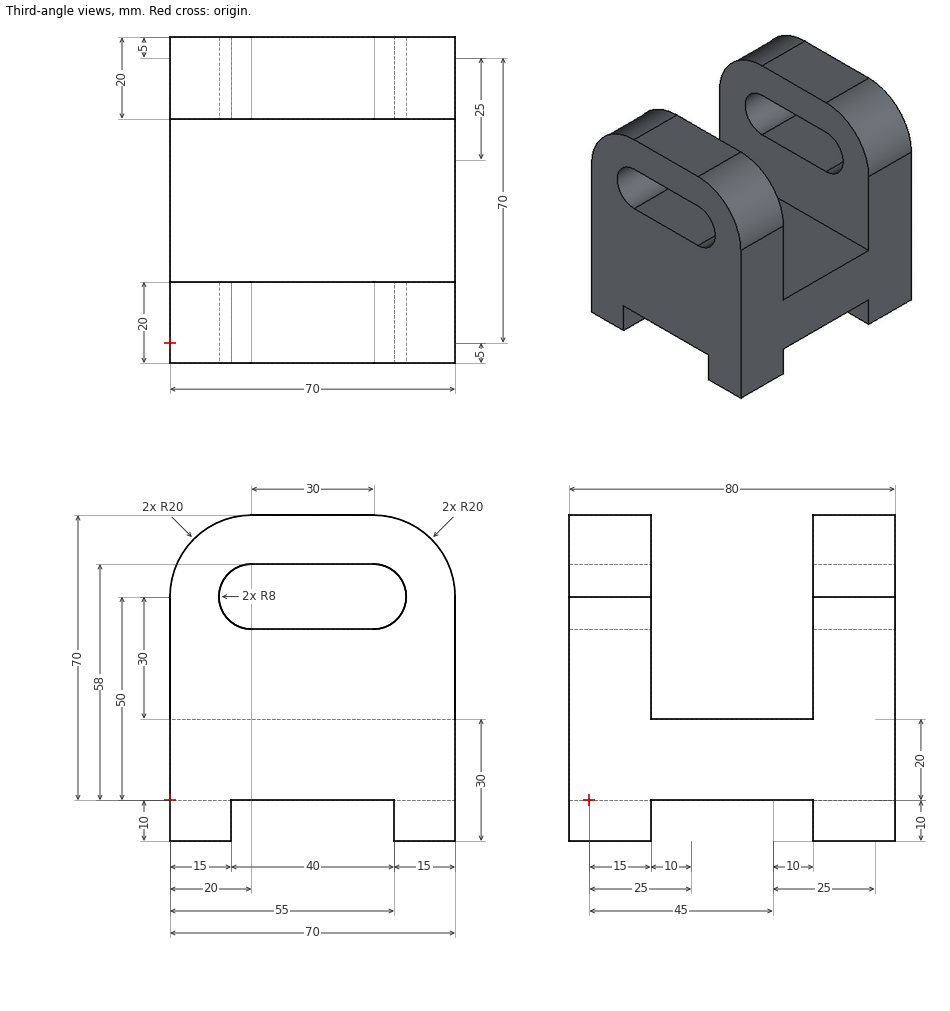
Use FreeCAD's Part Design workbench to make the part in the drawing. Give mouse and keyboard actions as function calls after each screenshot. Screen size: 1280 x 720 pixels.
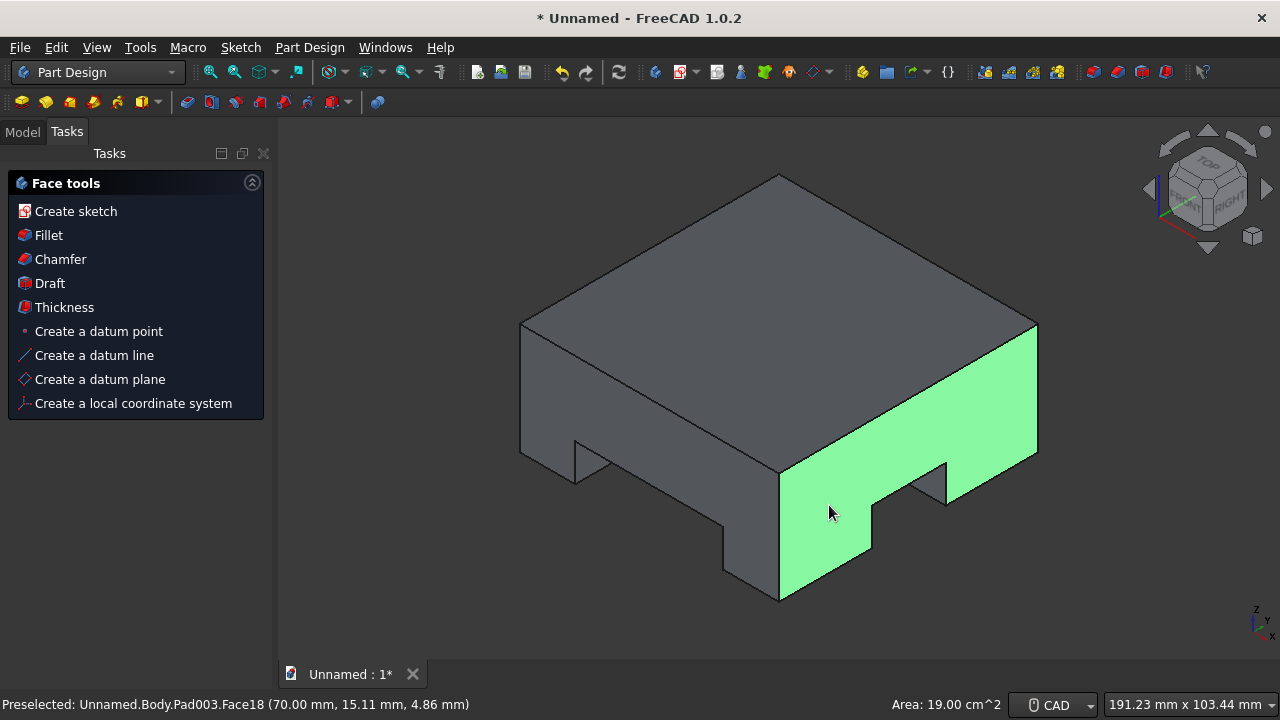
click(680, 72)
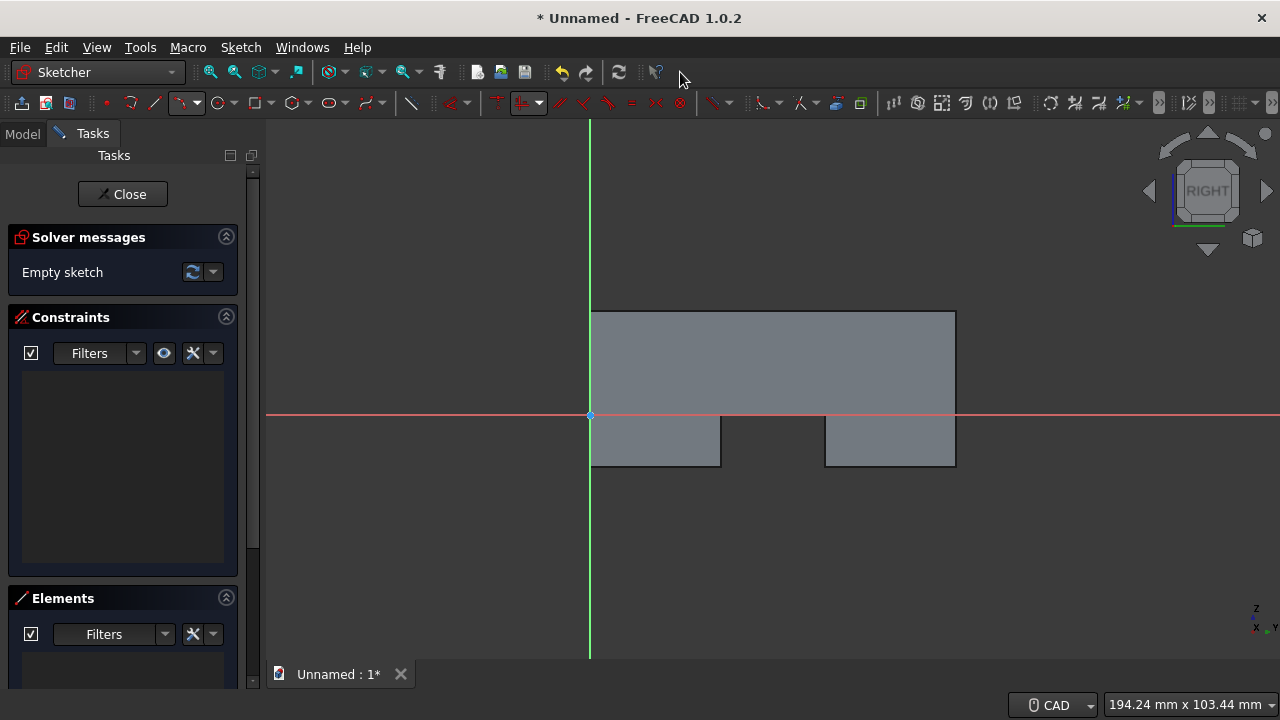
scroll(880, 452, up, 9)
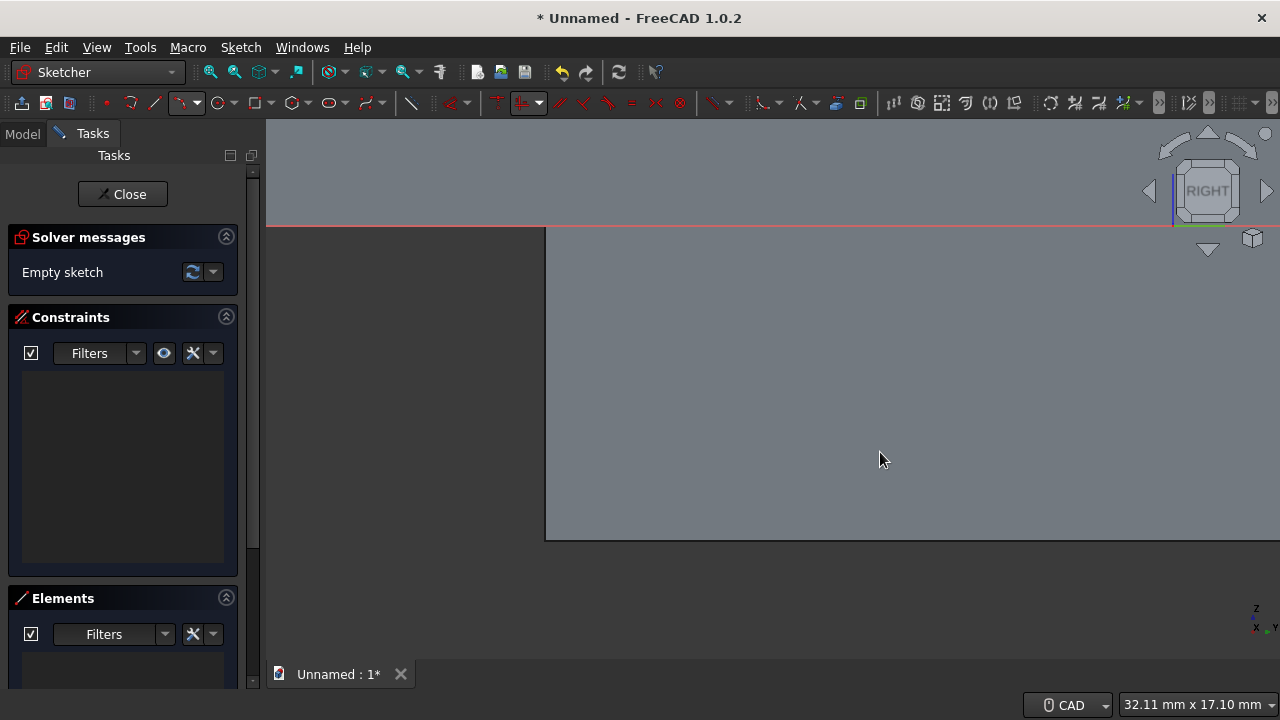
key(g)
key(r)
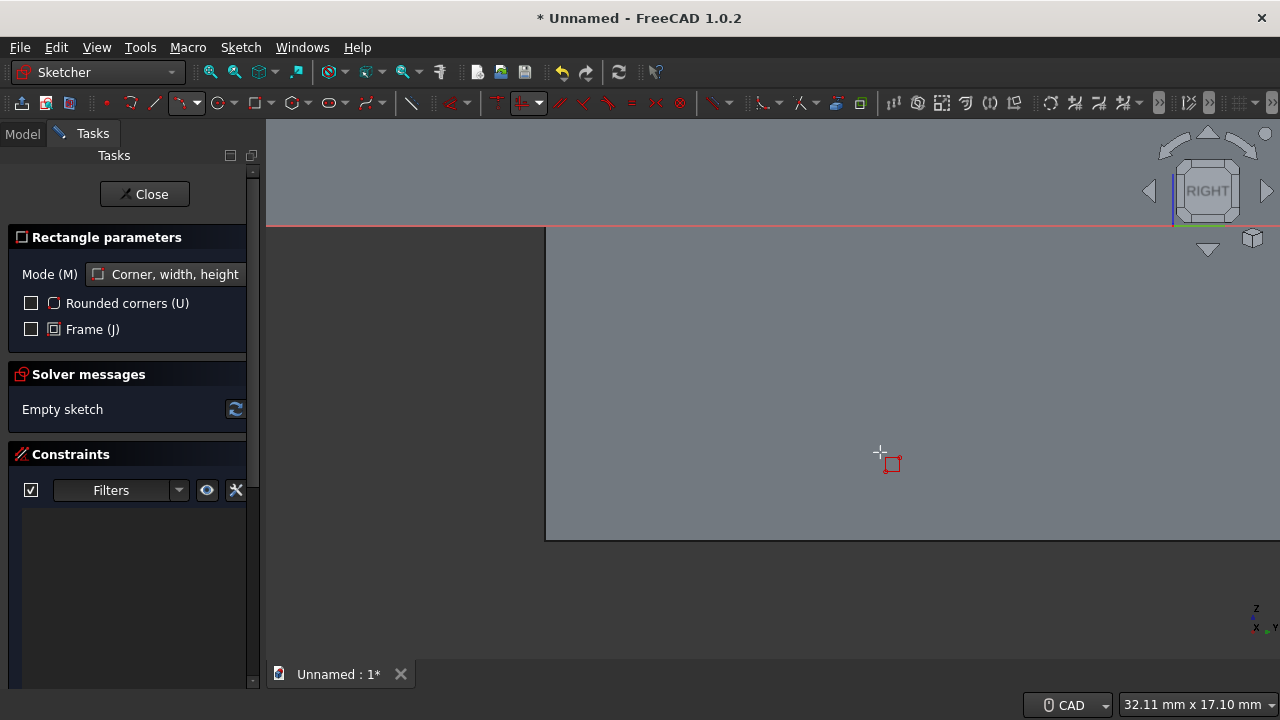
click(545, 226)
click(861, 541)
key(Escape)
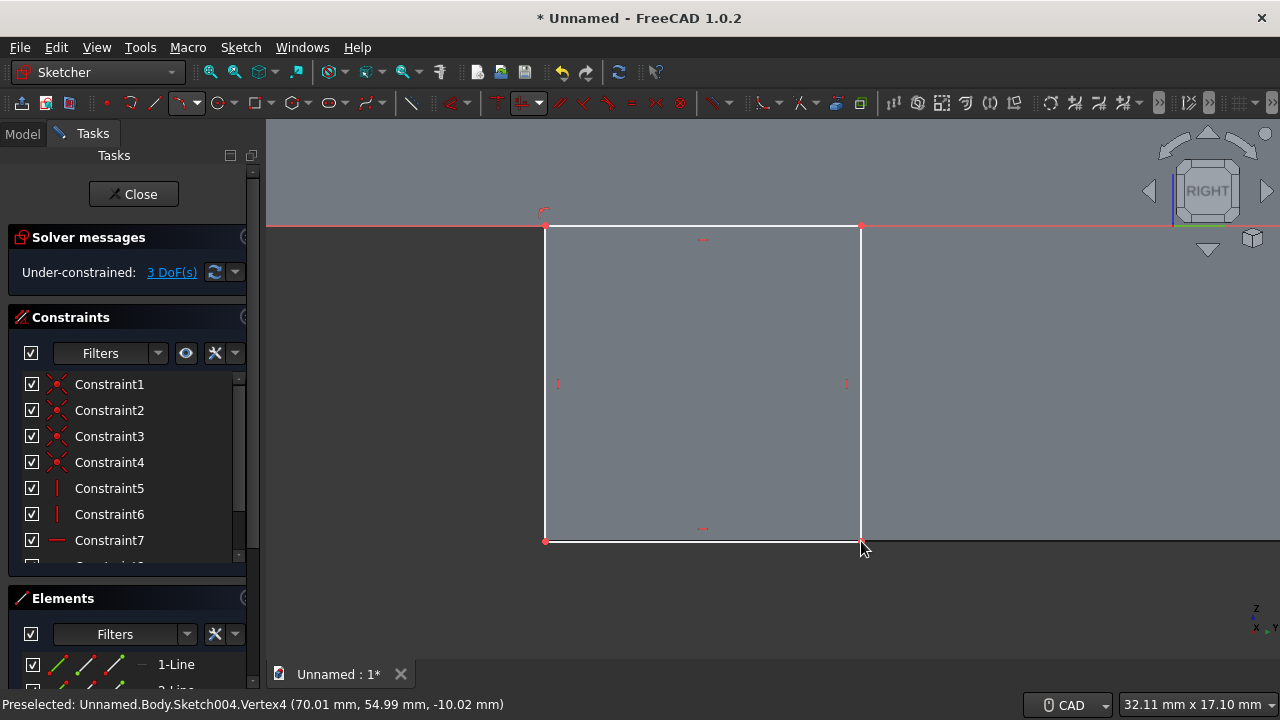
key(d)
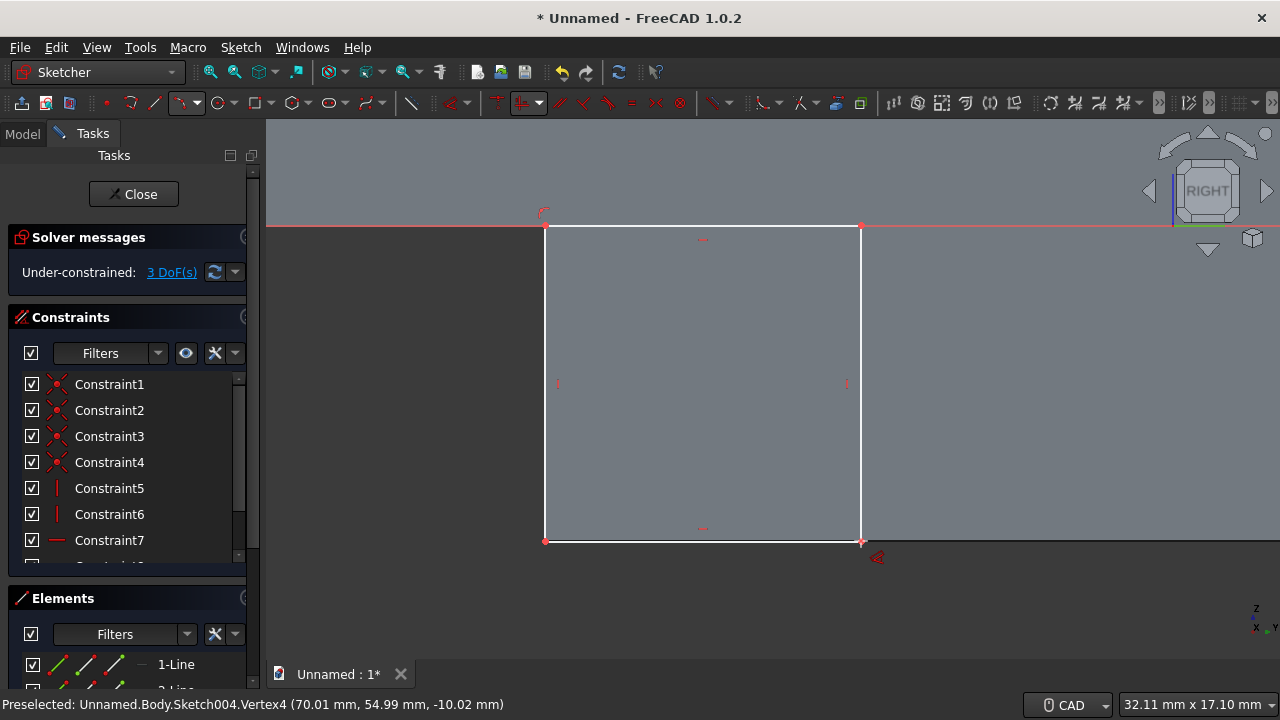
click(545, 321)
click(511, 384)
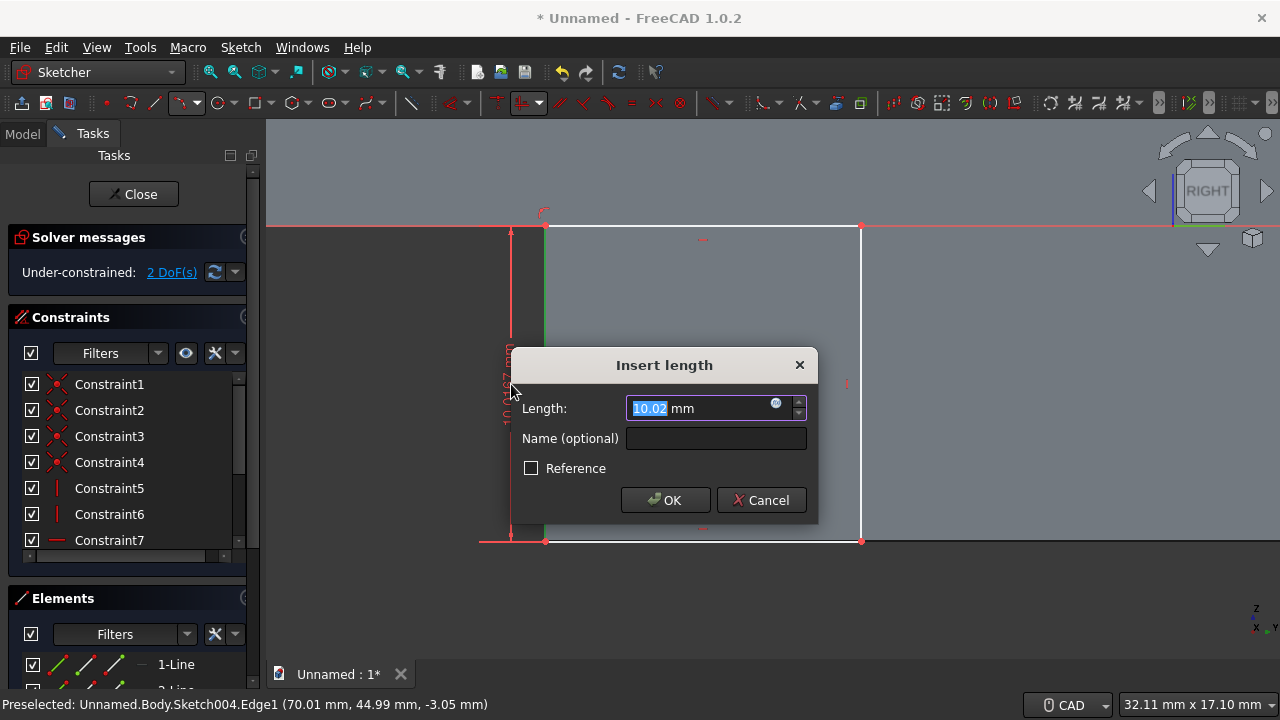
text(10)
key(Return)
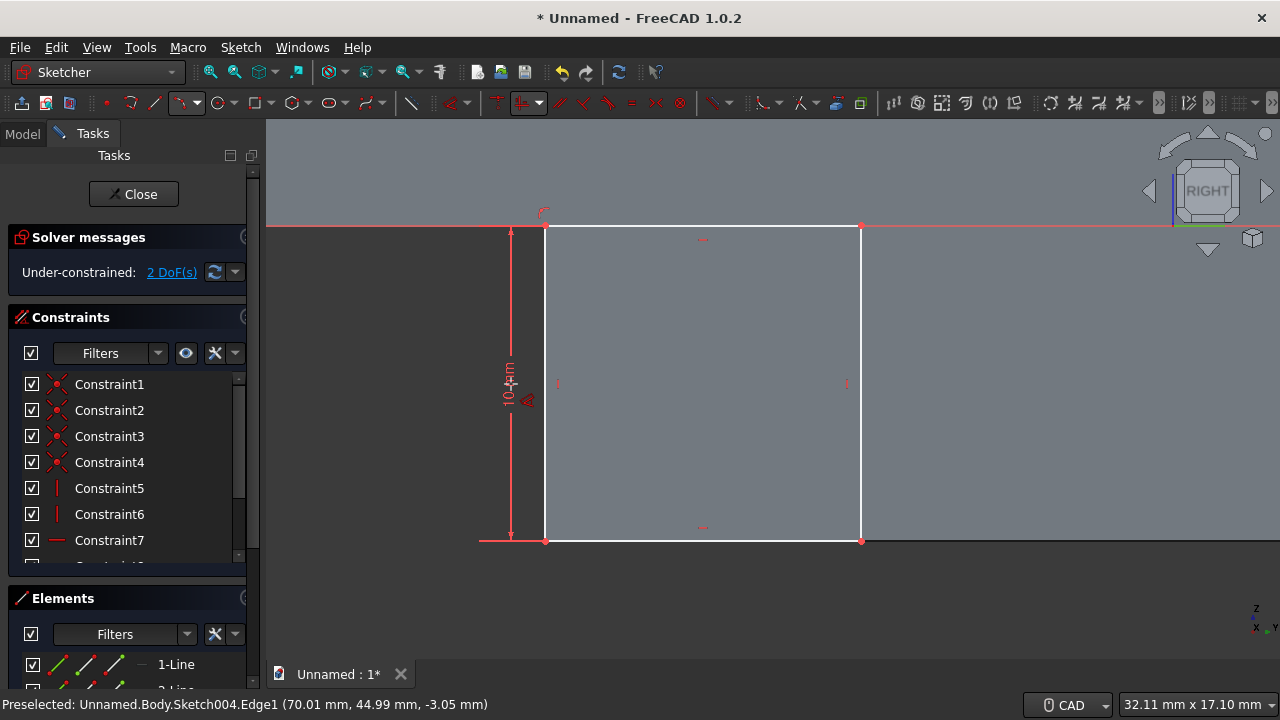
click(640, 541)
click(703, 575)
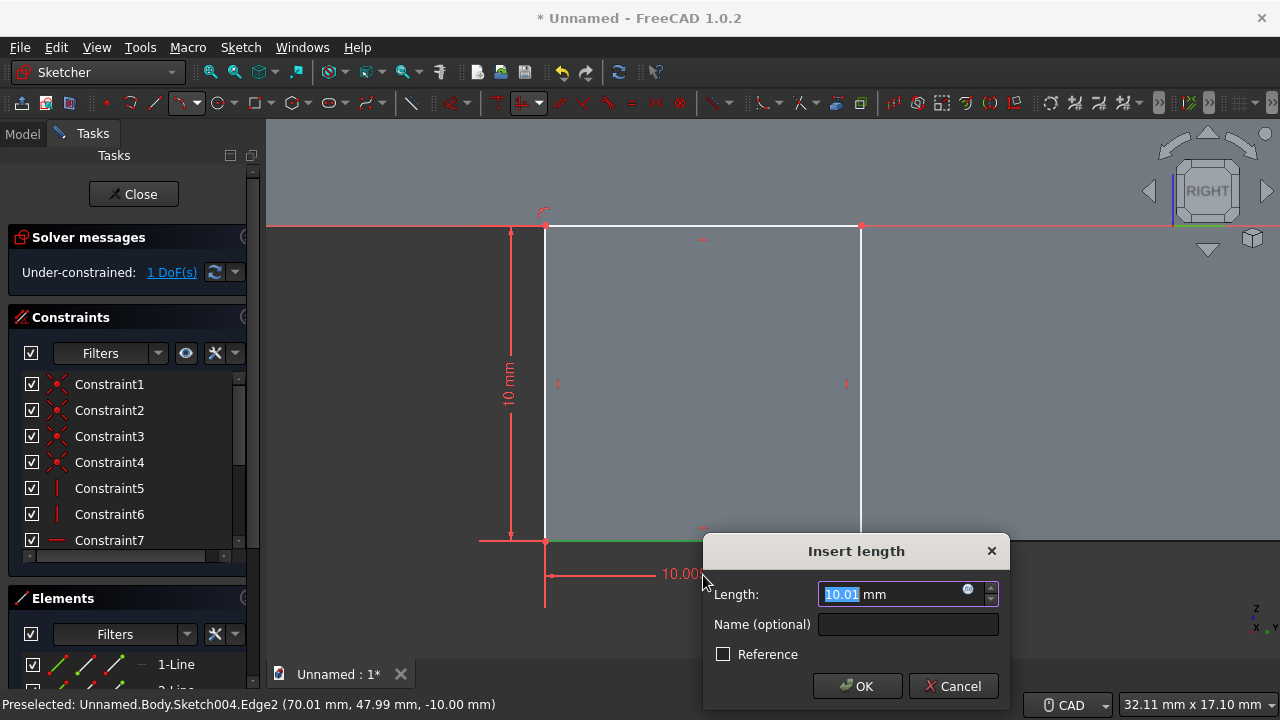
text(10)
key(Return)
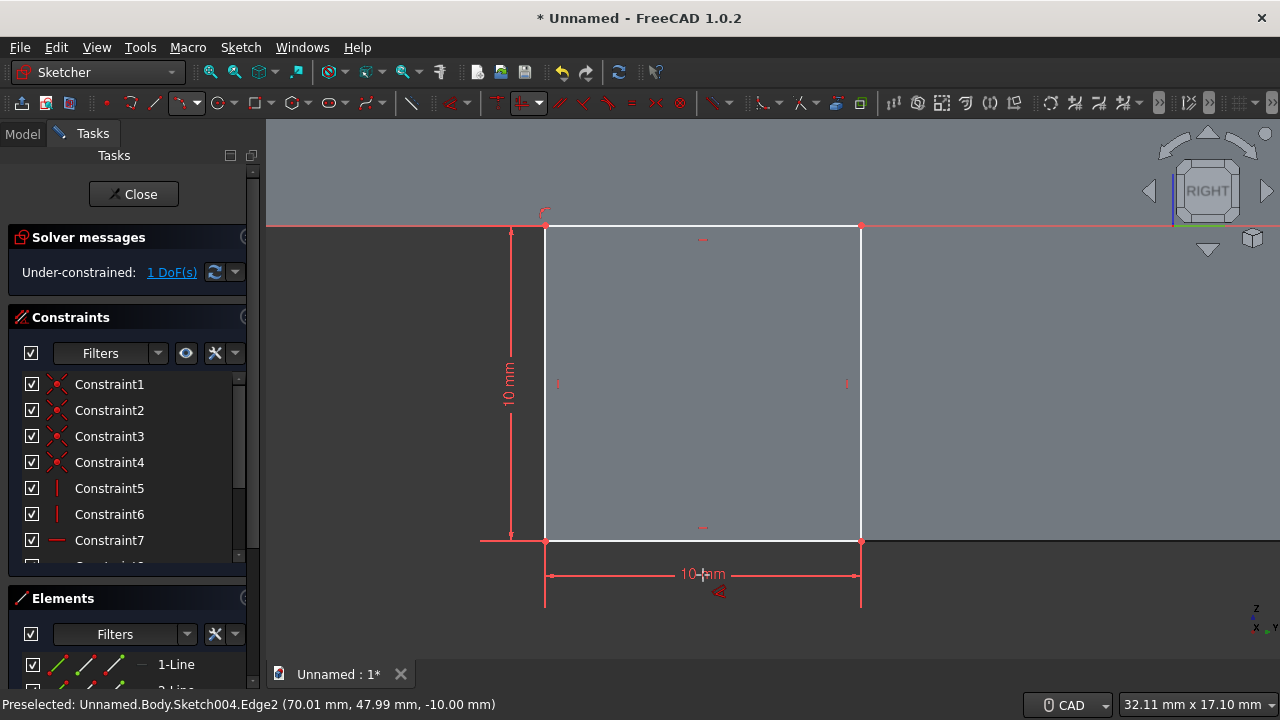
click(545, 226)
click(420, 192)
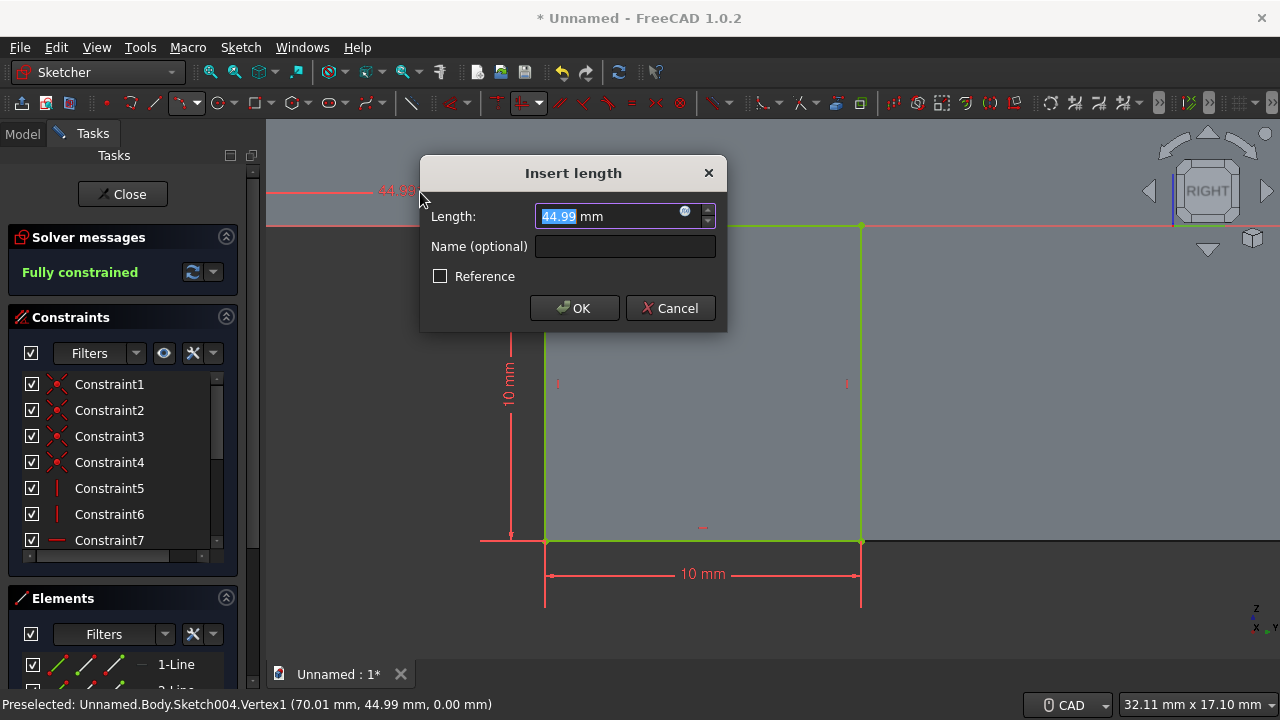
text(45)
key(Return)
key(Escape)